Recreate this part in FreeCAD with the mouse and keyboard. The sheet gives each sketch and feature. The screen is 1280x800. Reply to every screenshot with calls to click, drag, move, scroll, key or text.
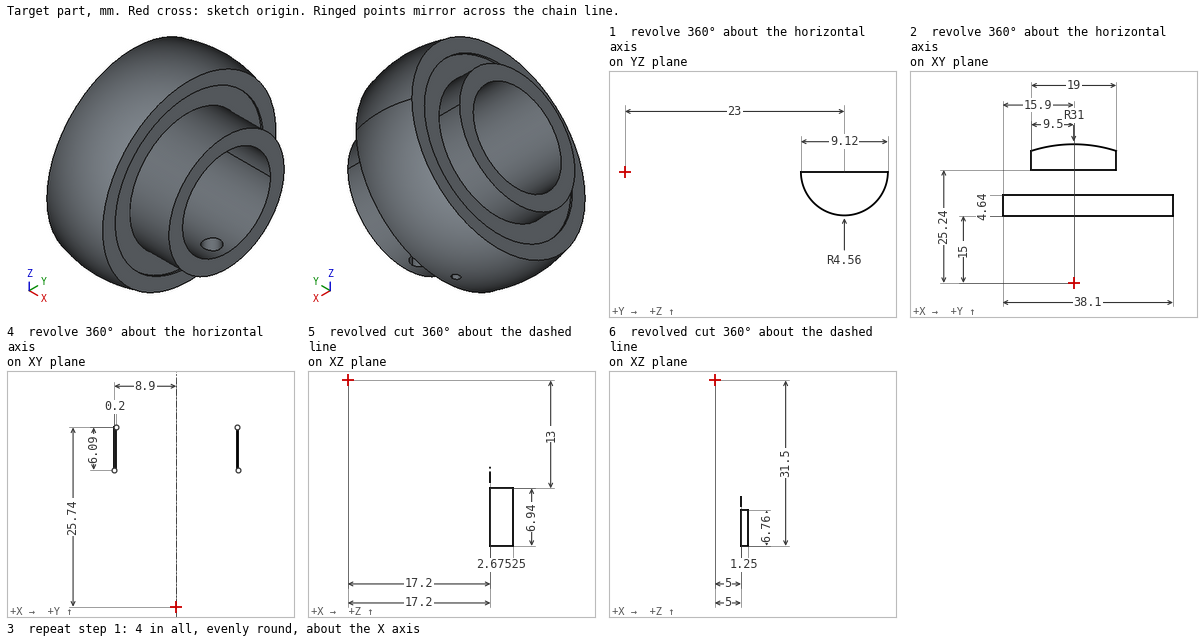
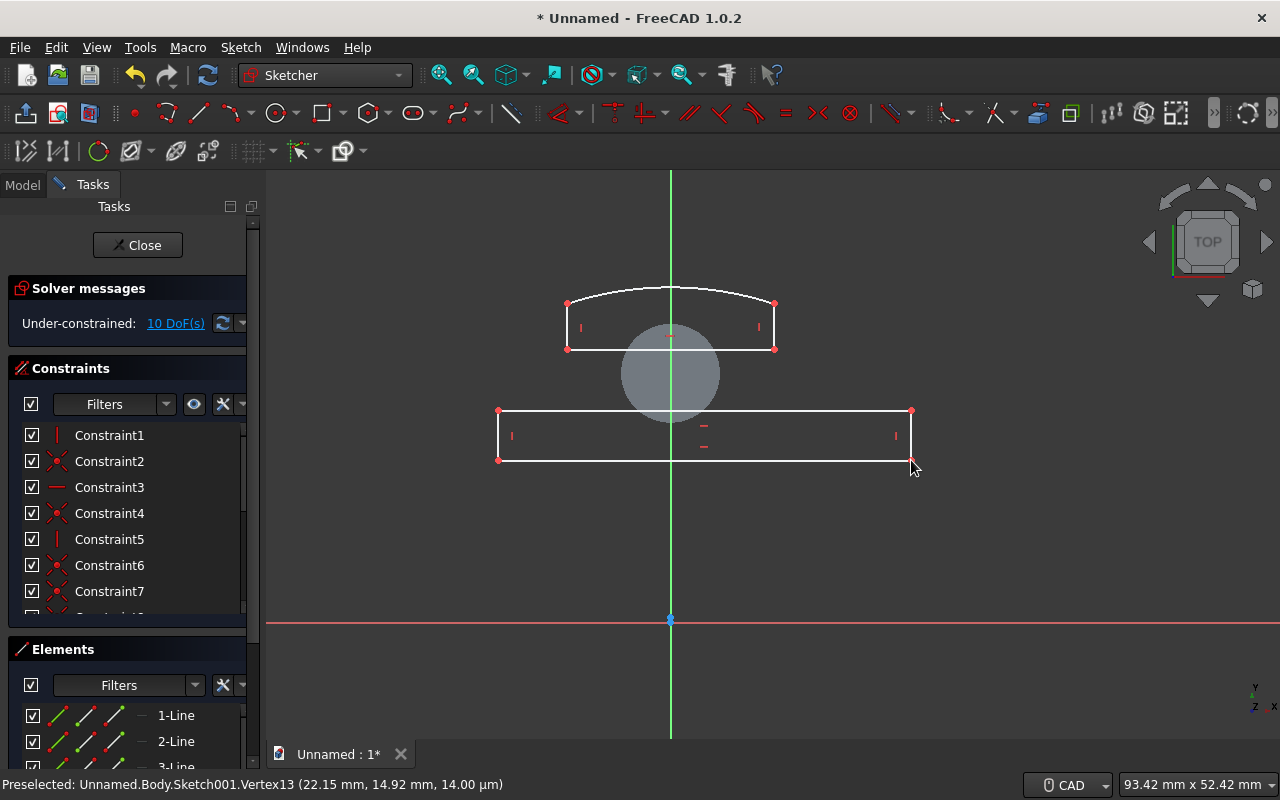
drag(661, 608, 681, 633)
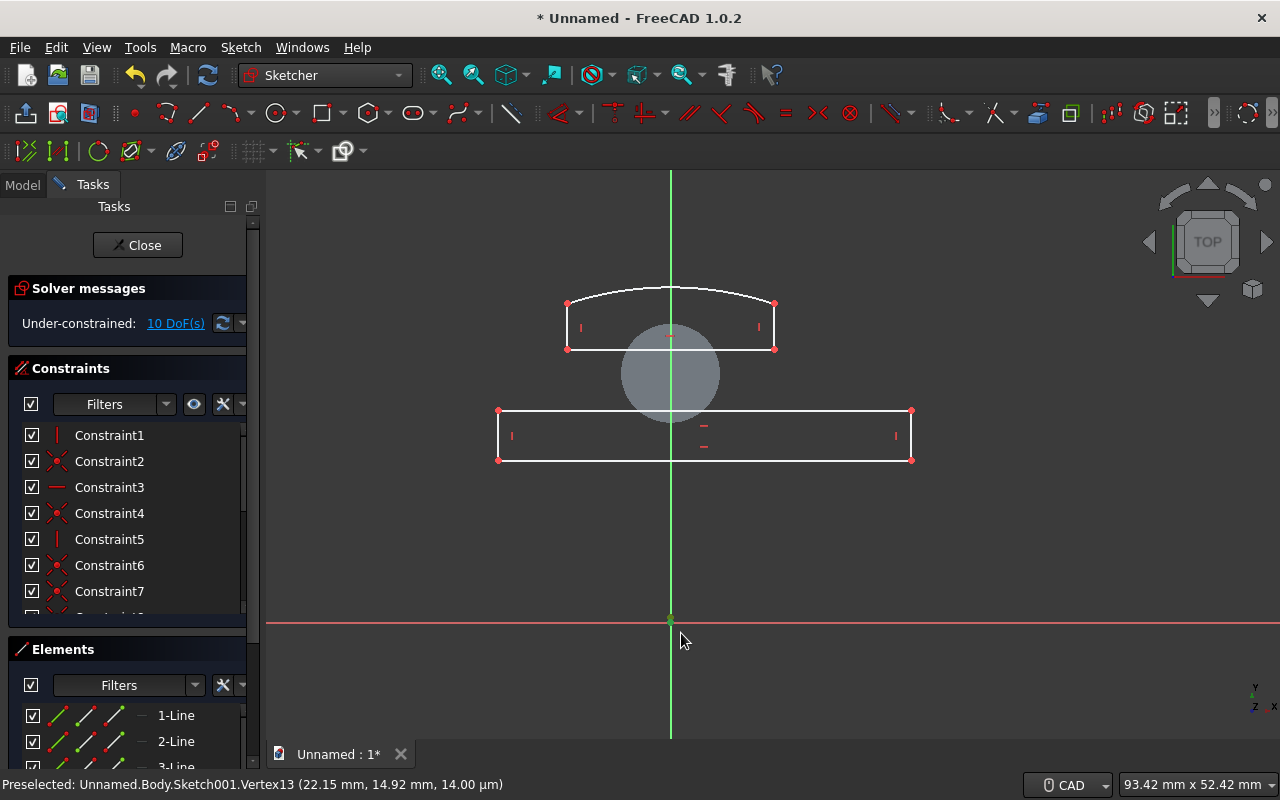
click(614, 114)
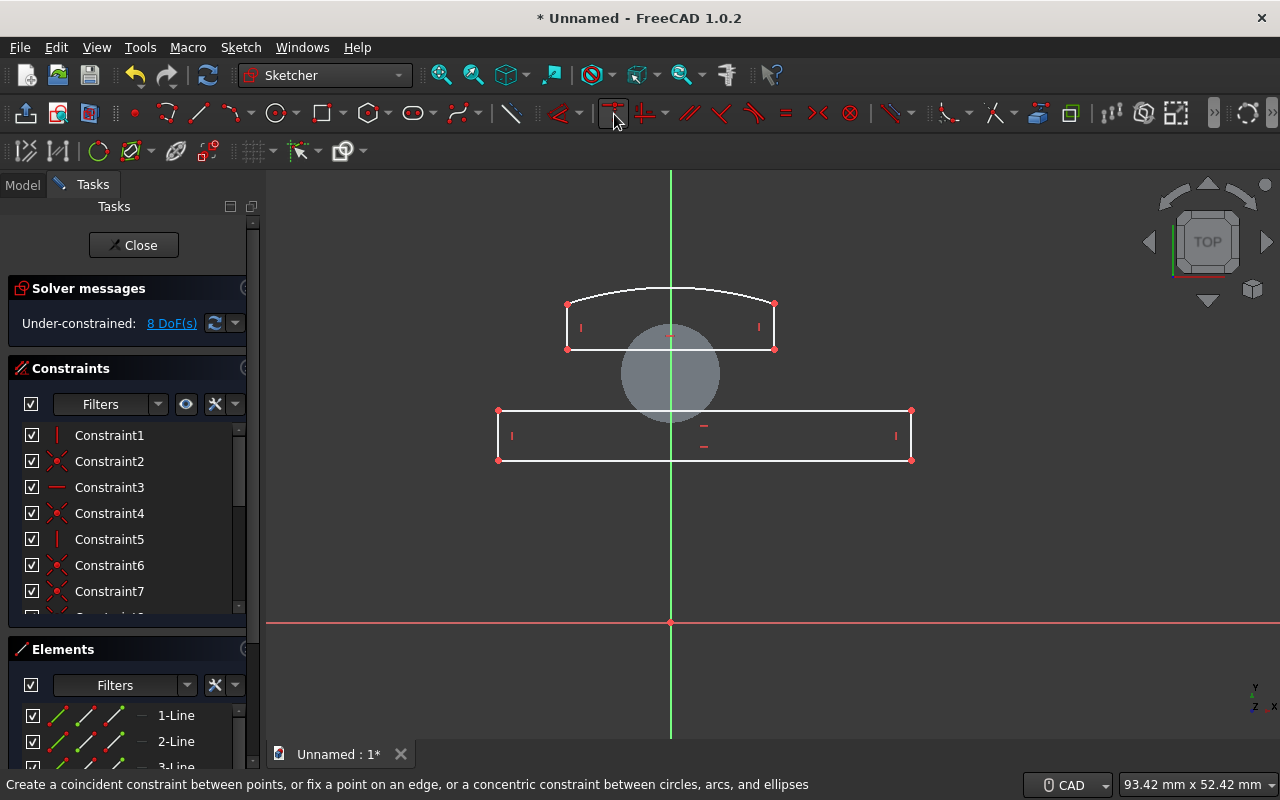
click(558, 114)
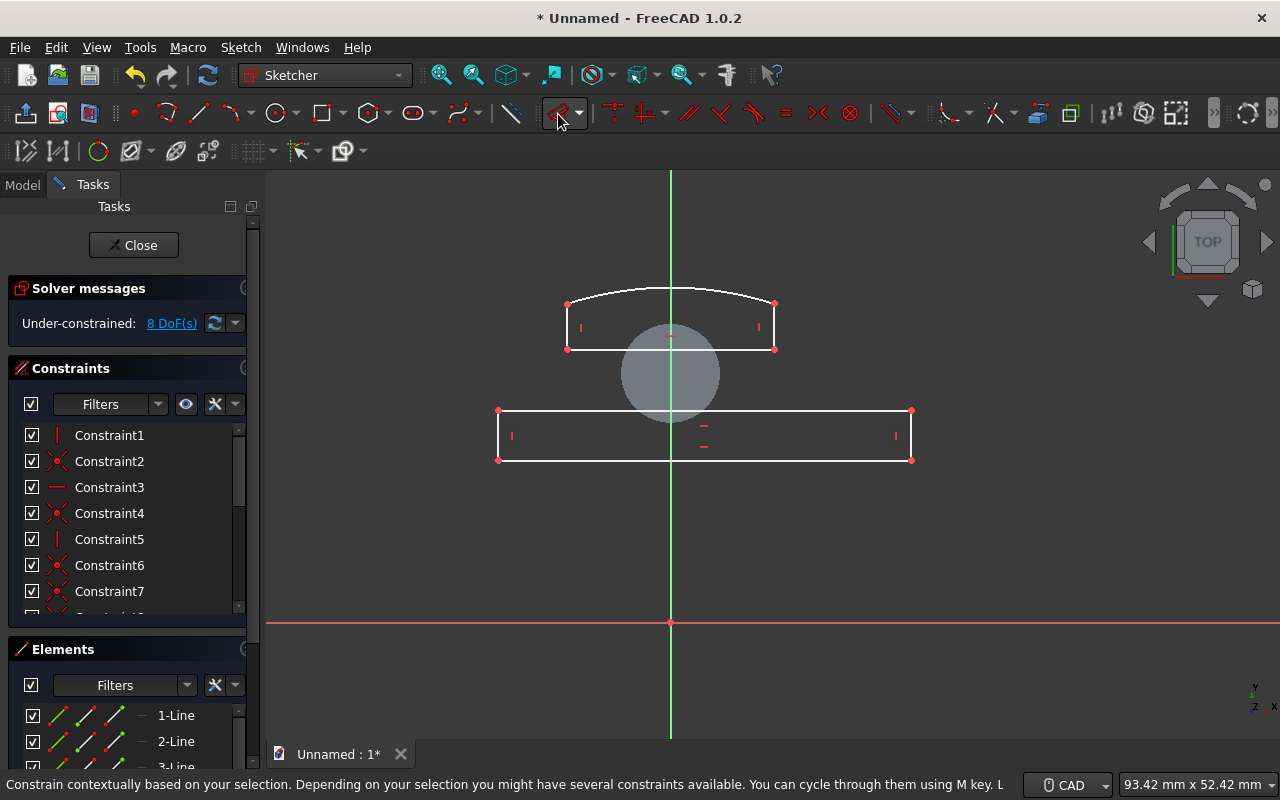
click(712, 290)
click(716, 258)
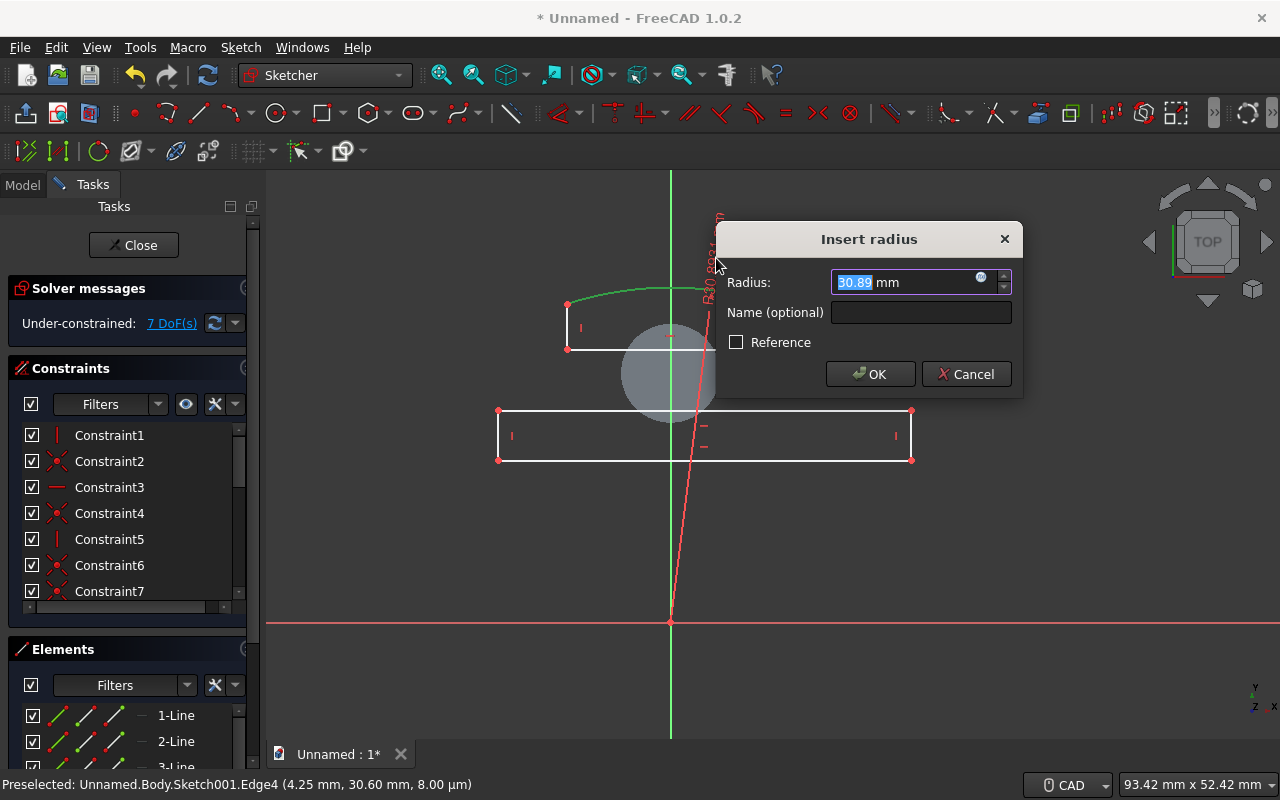
text(31)
key(Return)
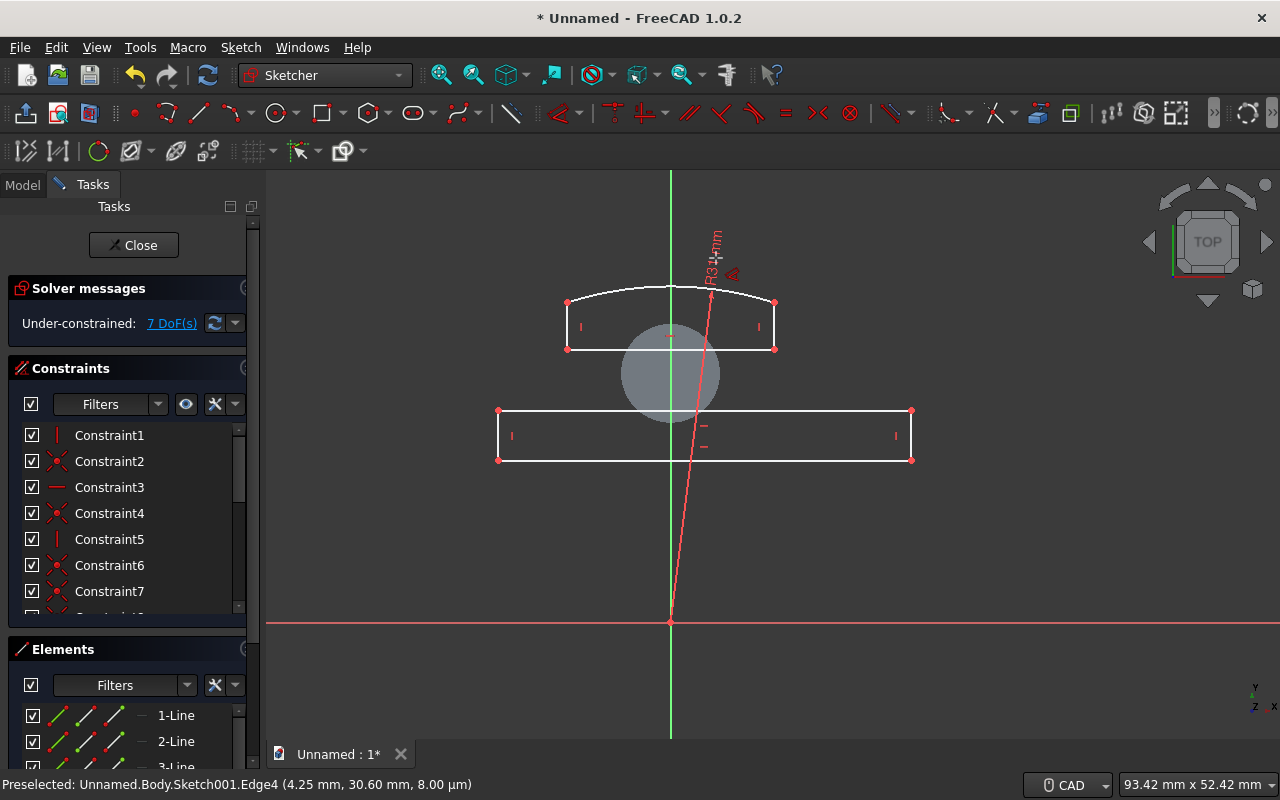
click(629, 350)
click(623, 316)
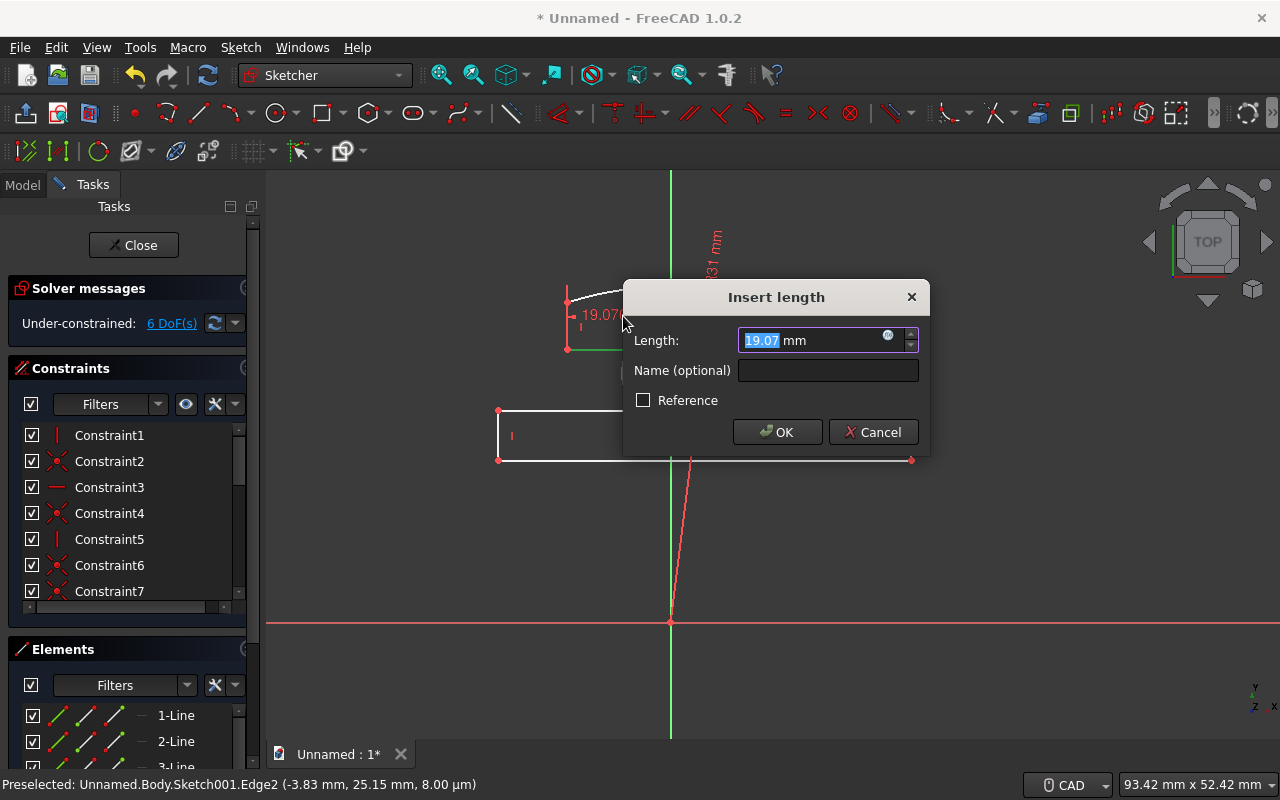
text(19)
key(Return)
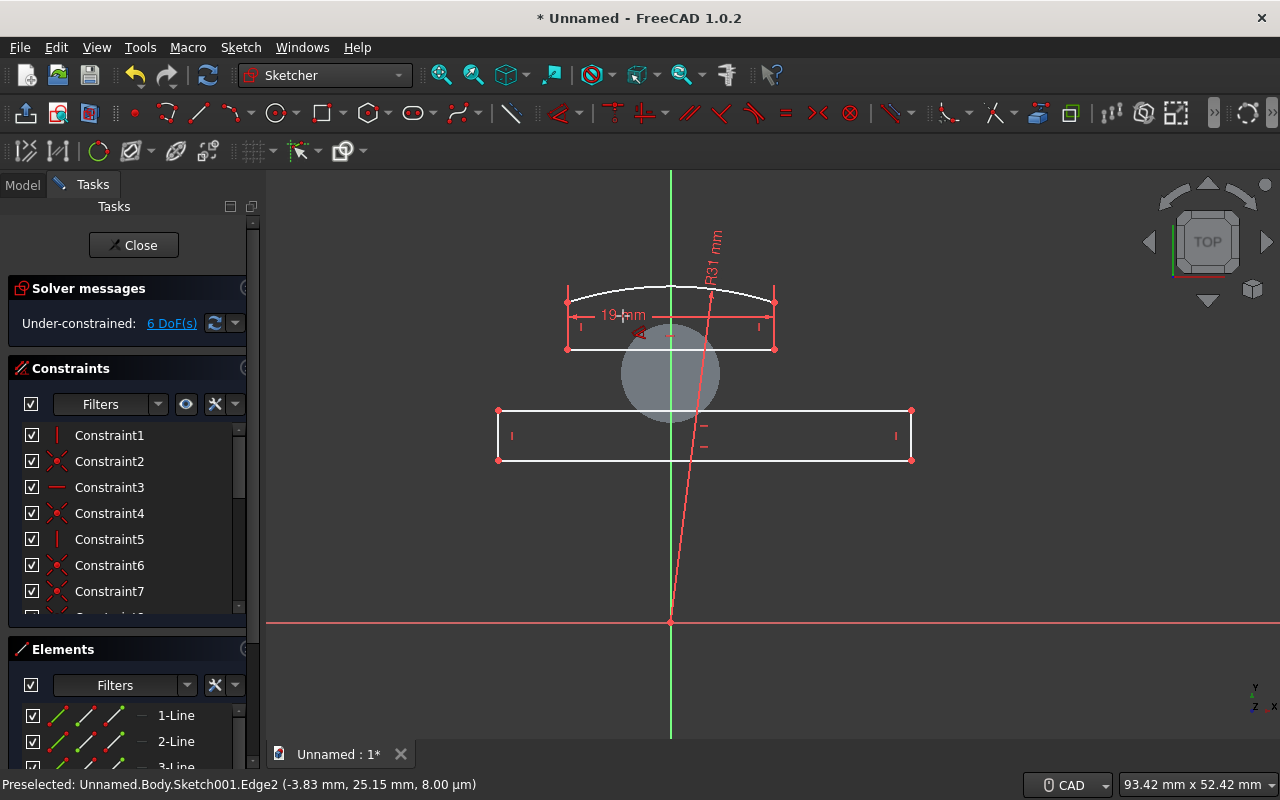
click(498, 461)
click(464, 542)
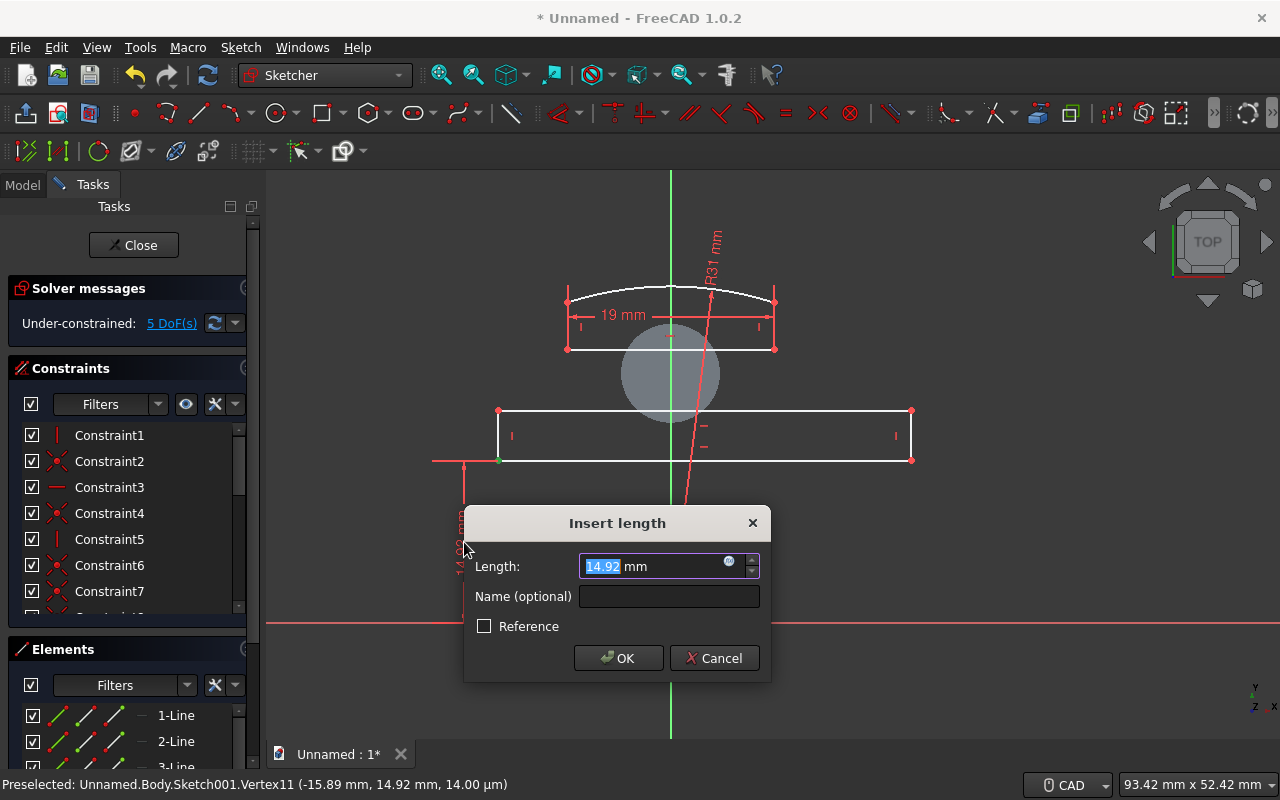
text(15)
key(Return)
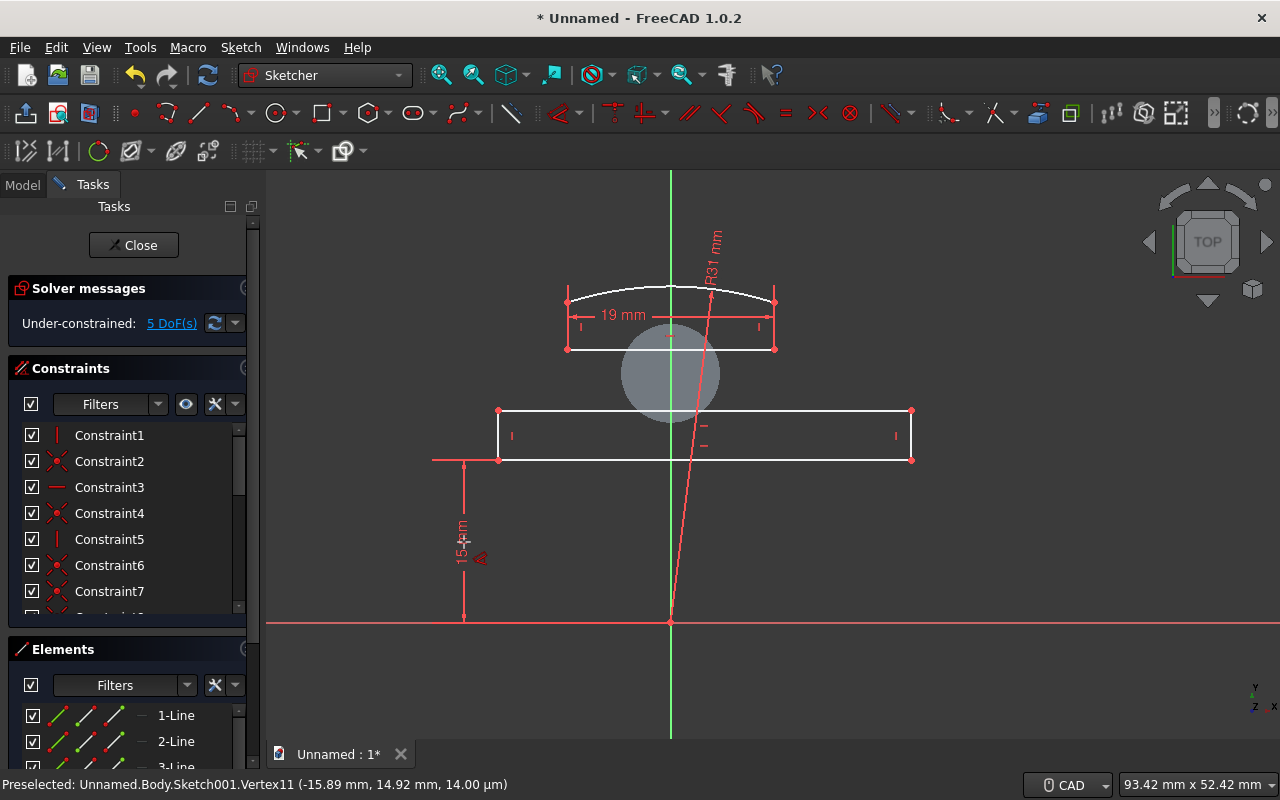
click(498, 426)
click(464, 436)